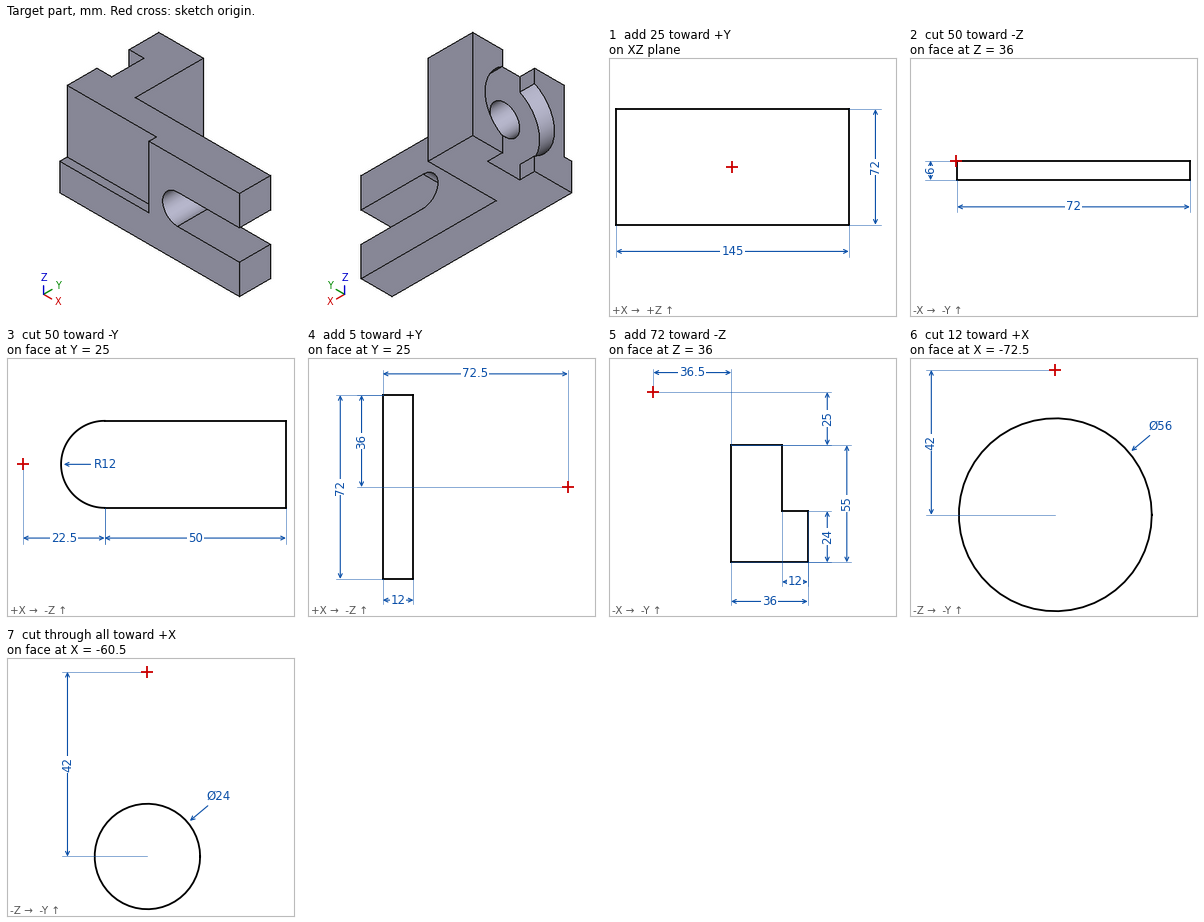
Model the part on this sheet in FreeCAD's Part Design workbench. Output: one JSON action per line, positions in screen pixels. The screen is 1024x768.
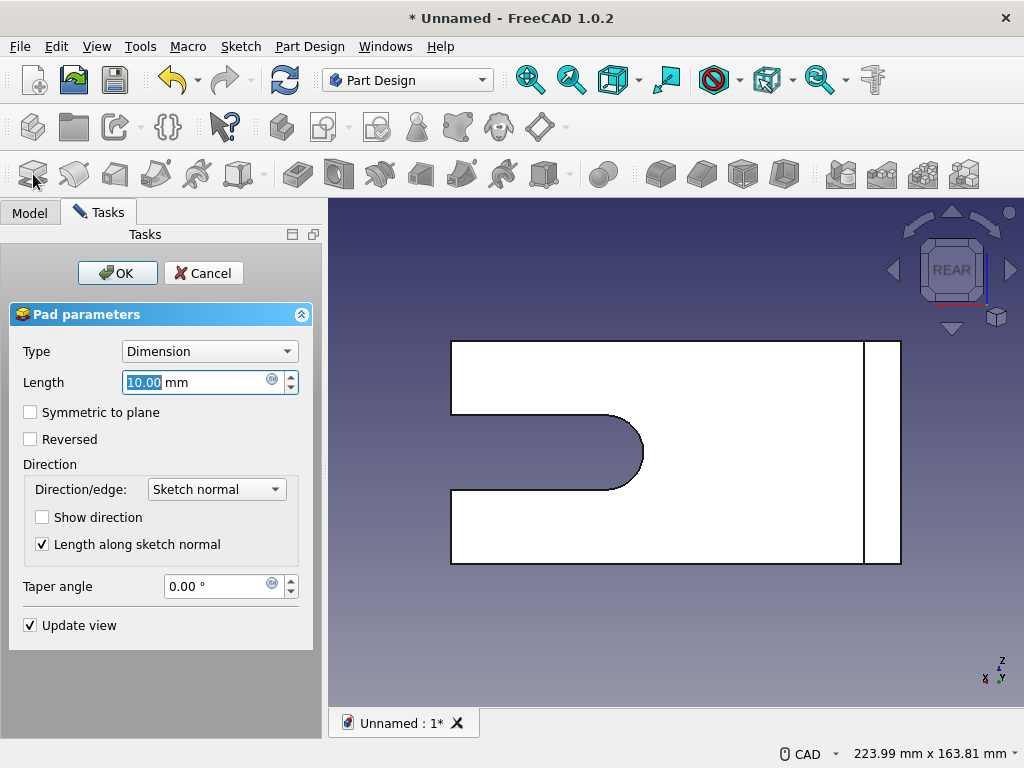
{"action": "type", "text": "5"}
{"action": "key", "text": "Tab"}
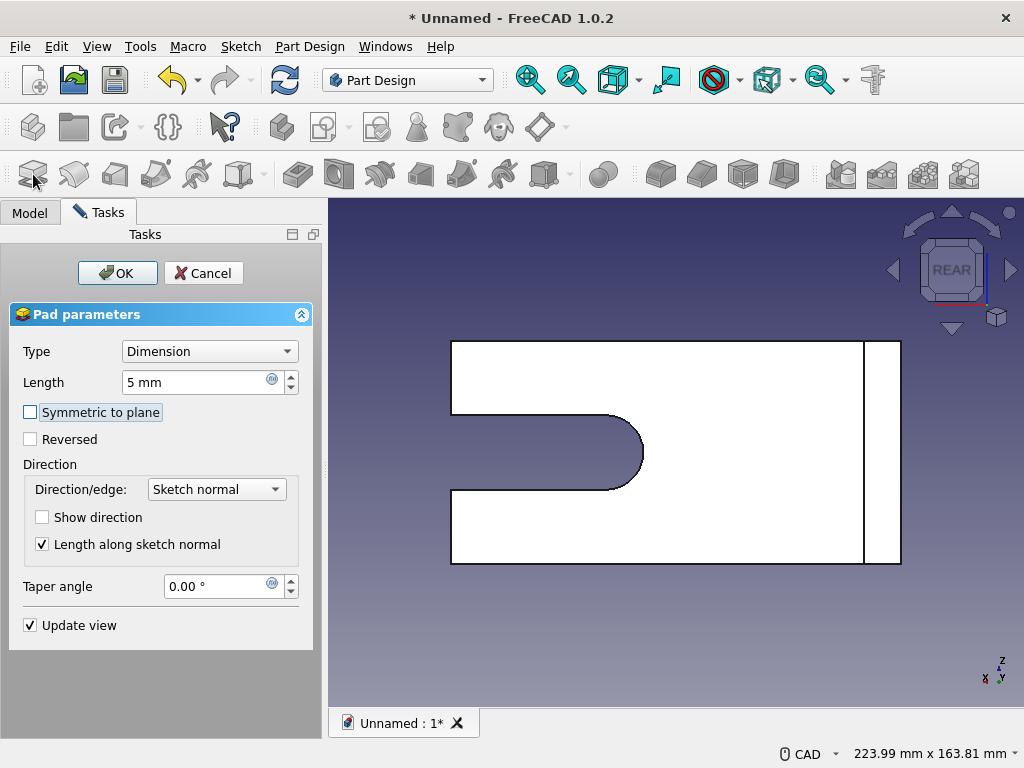
{"action": "left_click", "coordinate": [118, 273]}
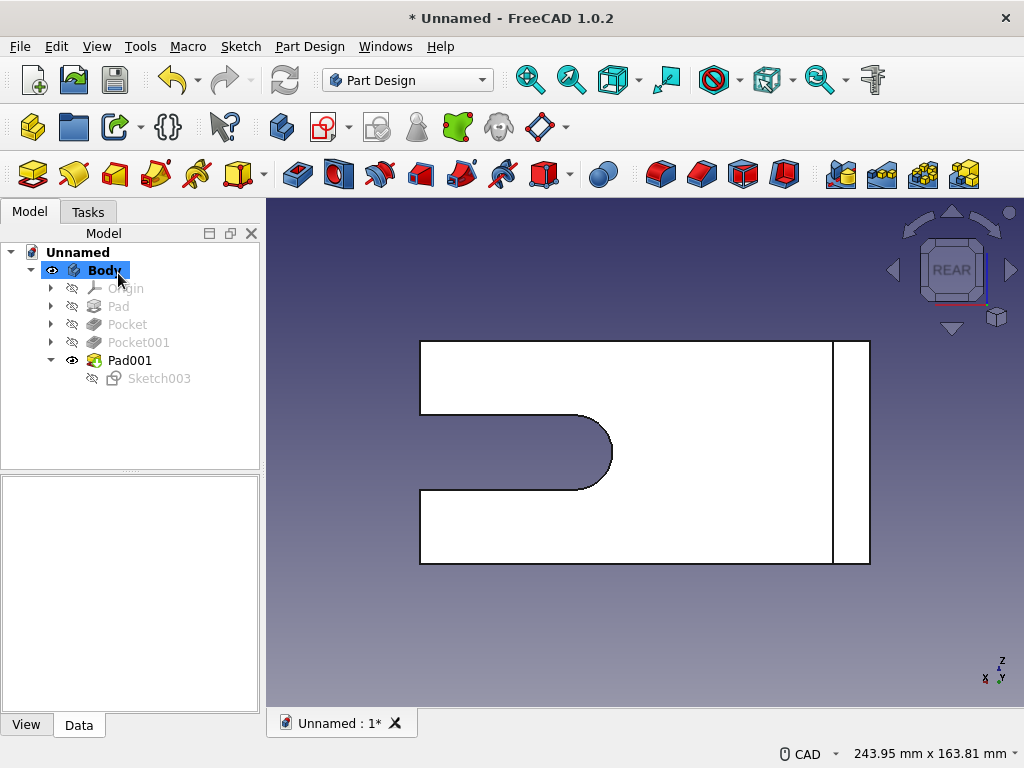
{"action": "key", "text": "0"}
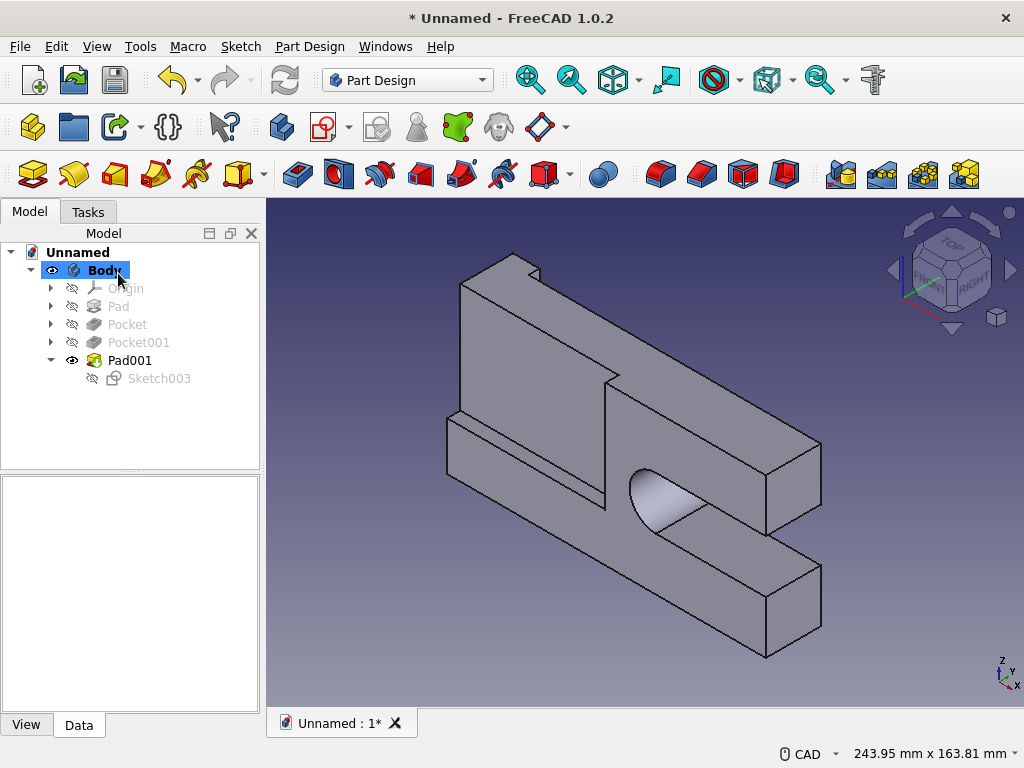
{"action": "left_click", "coordinate": [721, 421]}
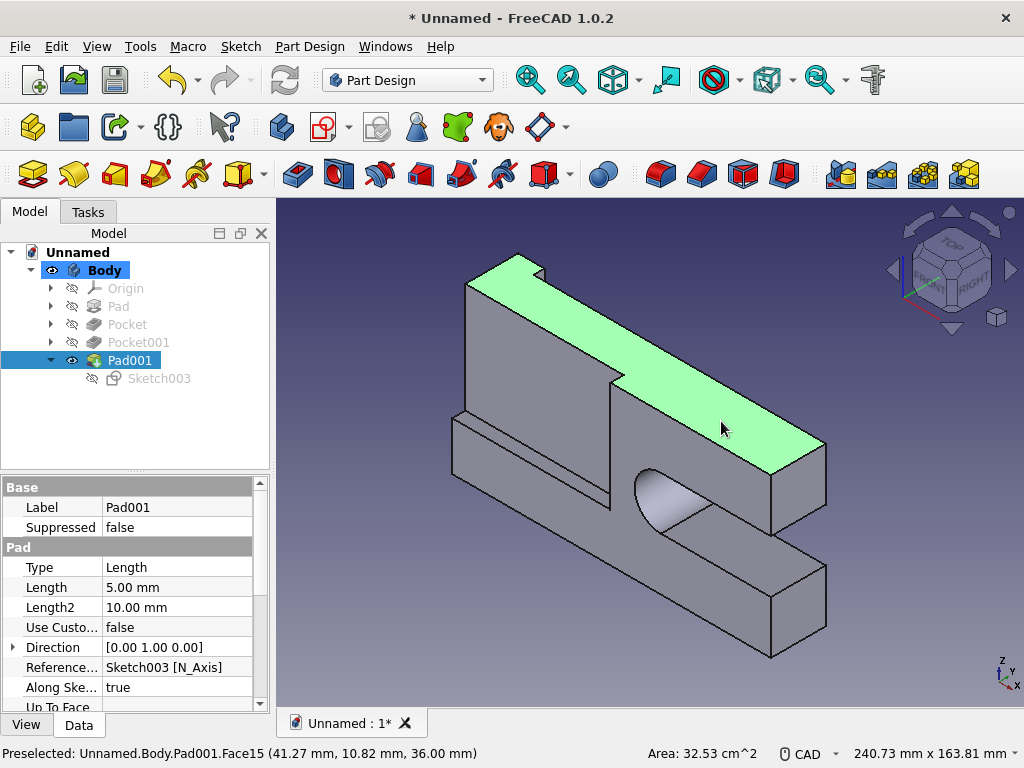
{"action": "left_click", "coordinate": [322, 128]}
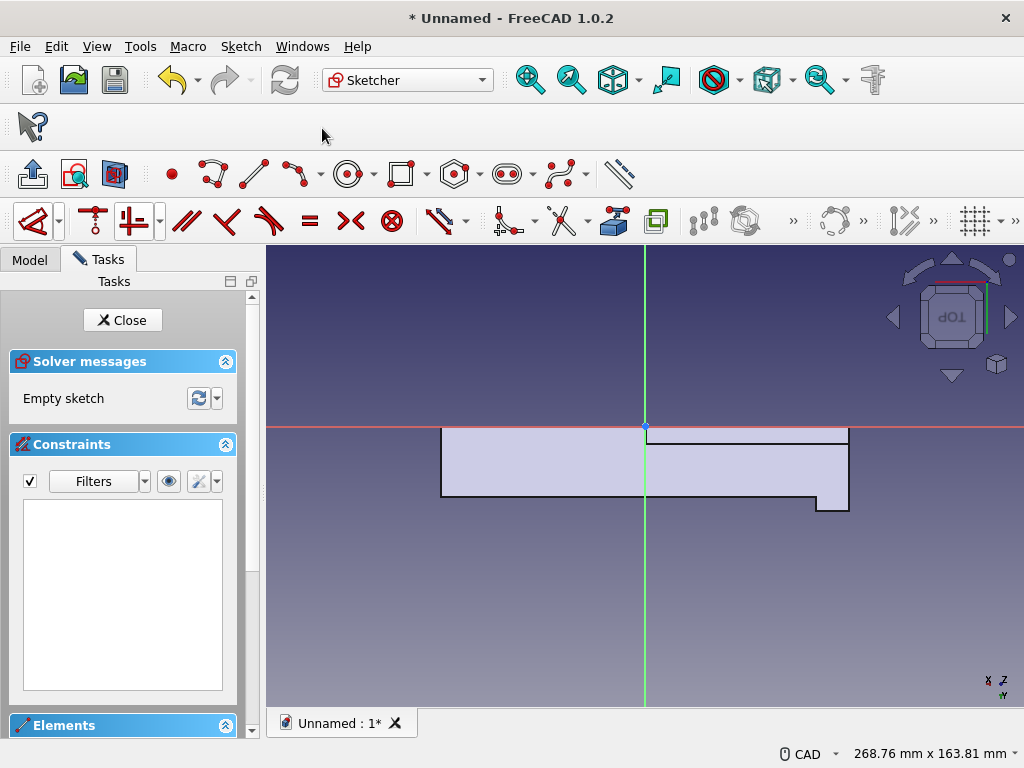
{"action": "scroll", "coordinate": [294, 273], "scroll_direction": "down", "scroll_amount": 1}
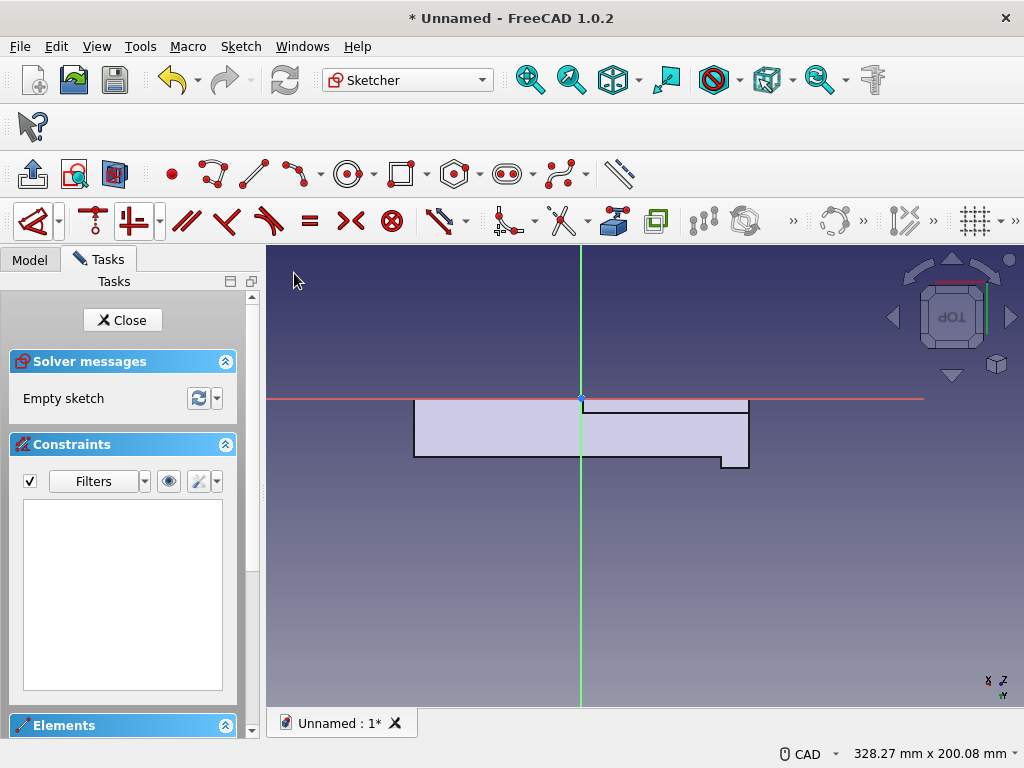
{"action": "scroll", "coordinate": [845, 522], "scroll_direction": "up", "scroll_amount": 2}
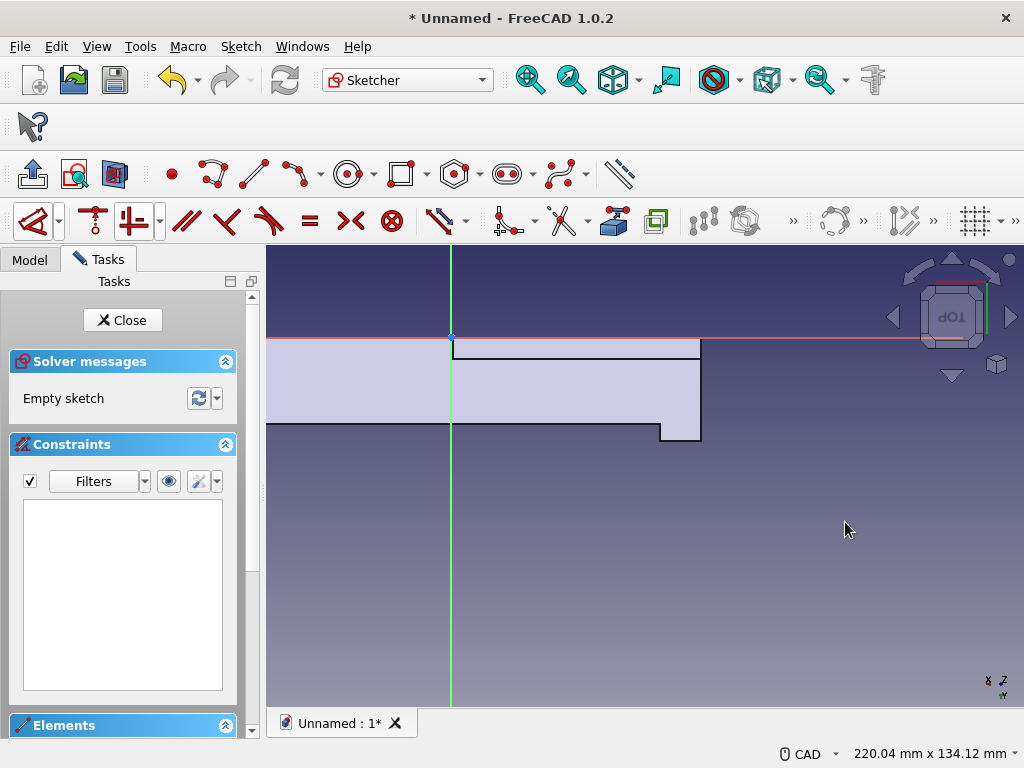
{"action": "left_click", "coordinate": [213, 174]}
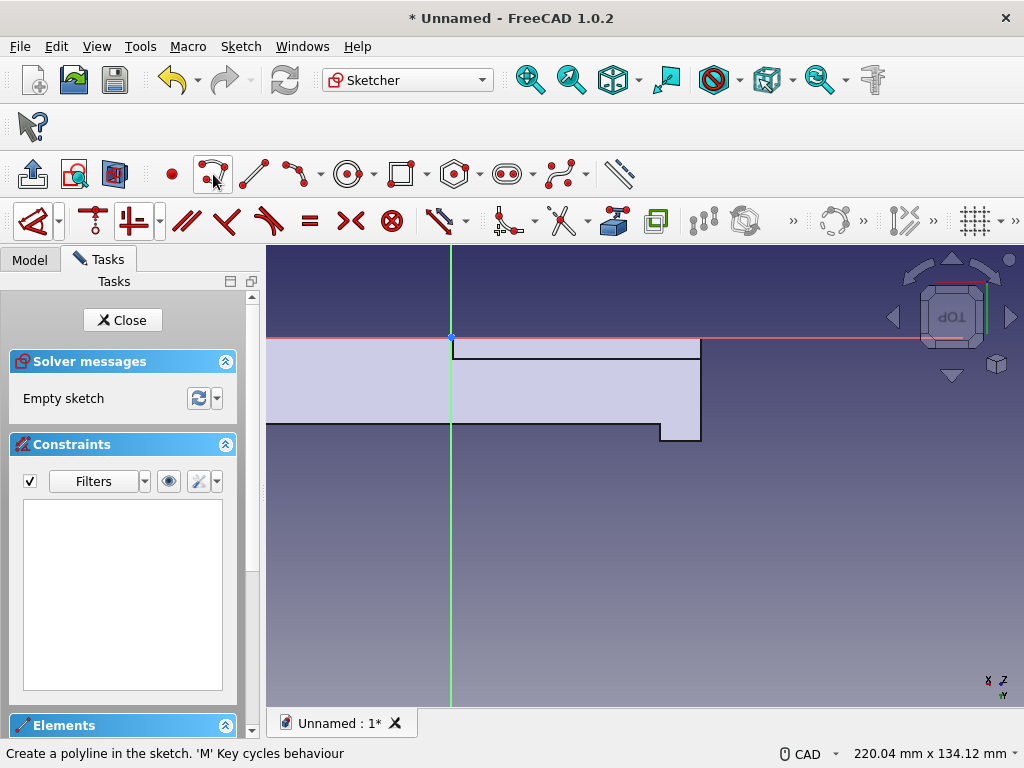
{"action": "left_click", "coordinate": [577, 424]}
{"action": "left_click", "coordinate": [577, 613]}
{"action": "left_click", "coordinate": [701, 613]}
{"action": "left_click", "coordinate": [701, 531]}
{"action": "left_click", "coordinate": [660, 531]}
{"action": "left_click", "coordinate": [660, 424]}
{"action": "left_click", "coordinate": [577, 425]}
{"action": "key", "text": "Escape"}
{"action": "key", "text": "Escape"}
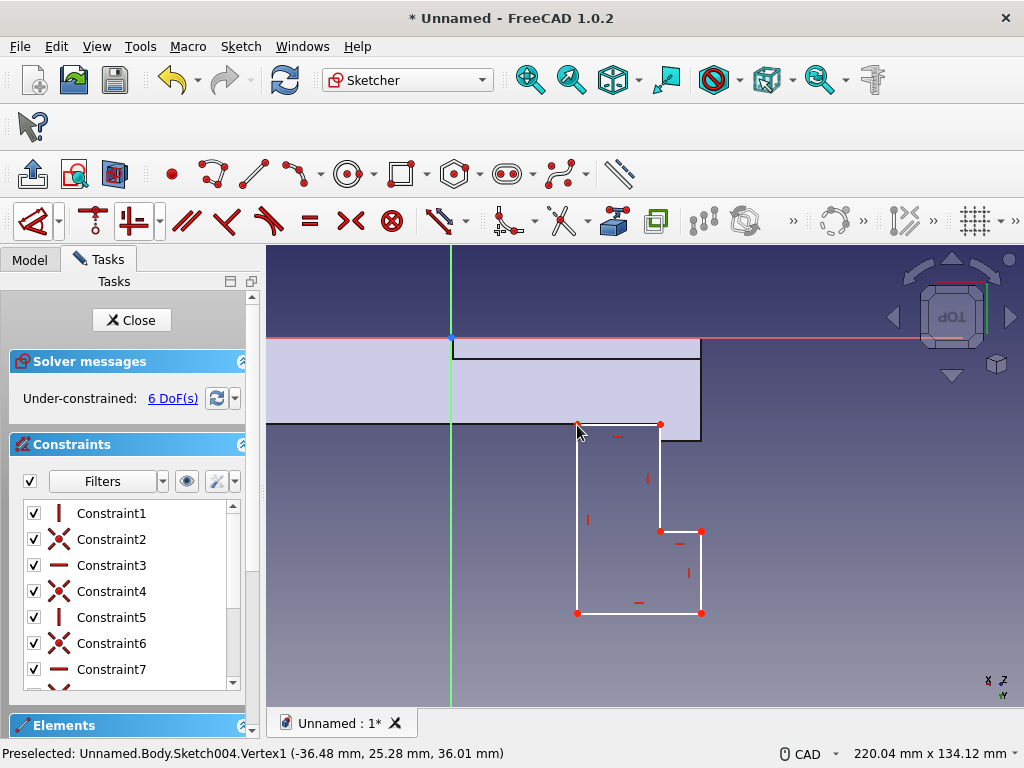
{"action": "left_click", "coordinate": [577, 482]}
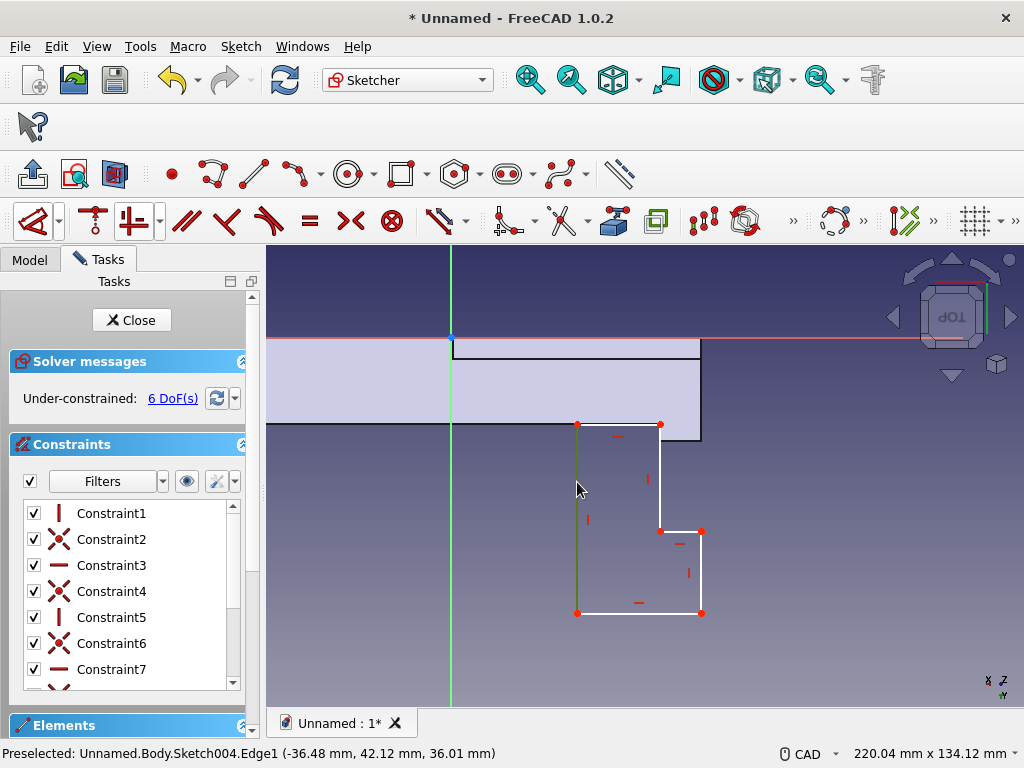
{"action": "left_click", "coordinate": [58, 222]}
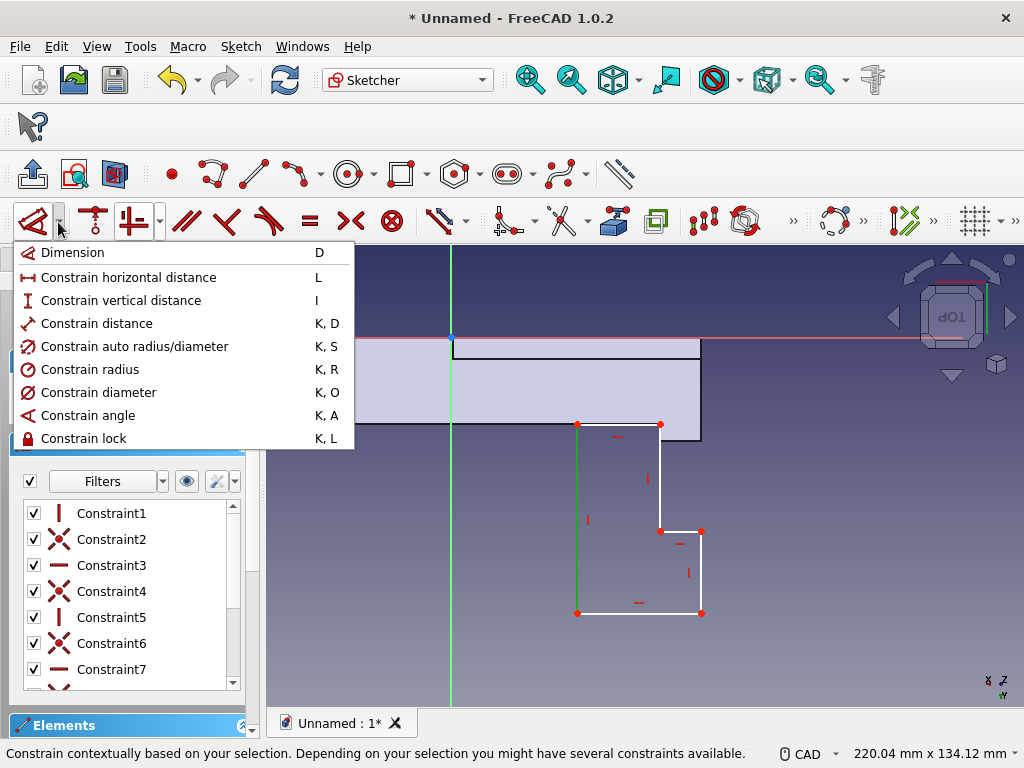
{"action": "left_click", "coordinate": [184, 300]}